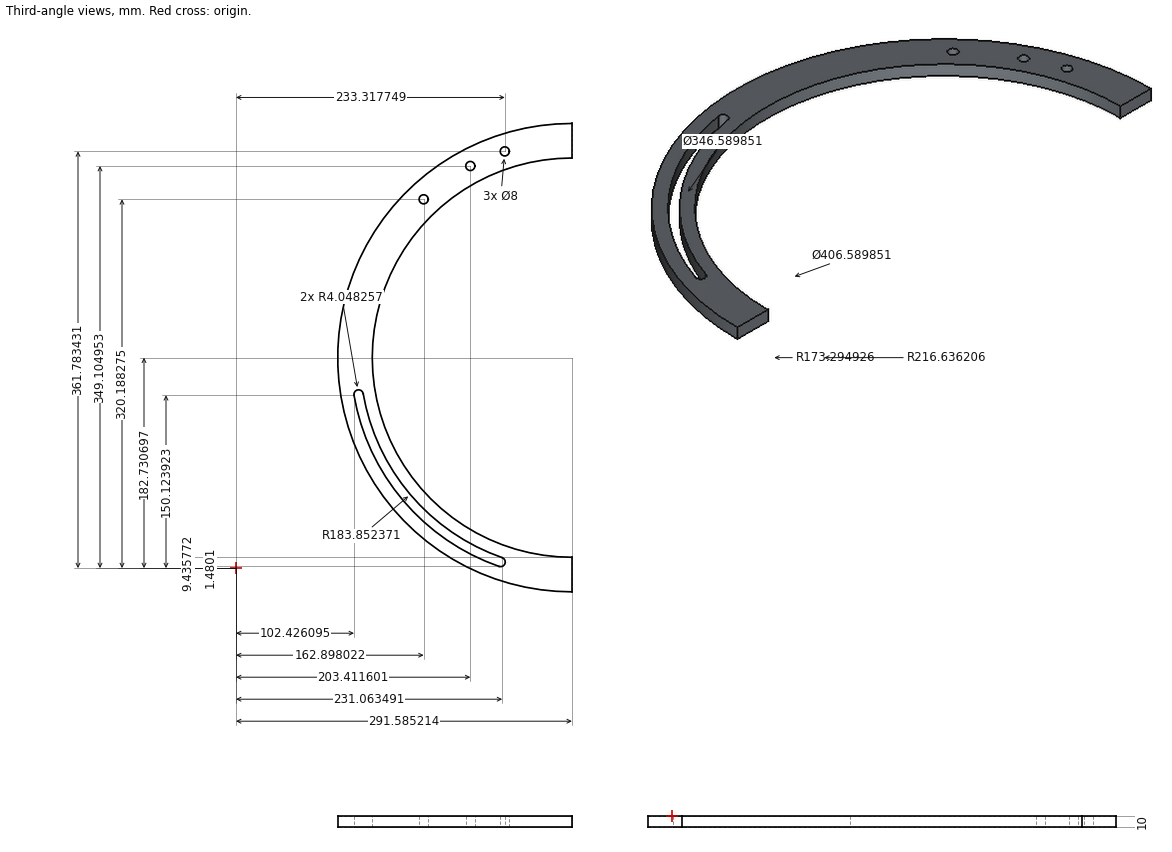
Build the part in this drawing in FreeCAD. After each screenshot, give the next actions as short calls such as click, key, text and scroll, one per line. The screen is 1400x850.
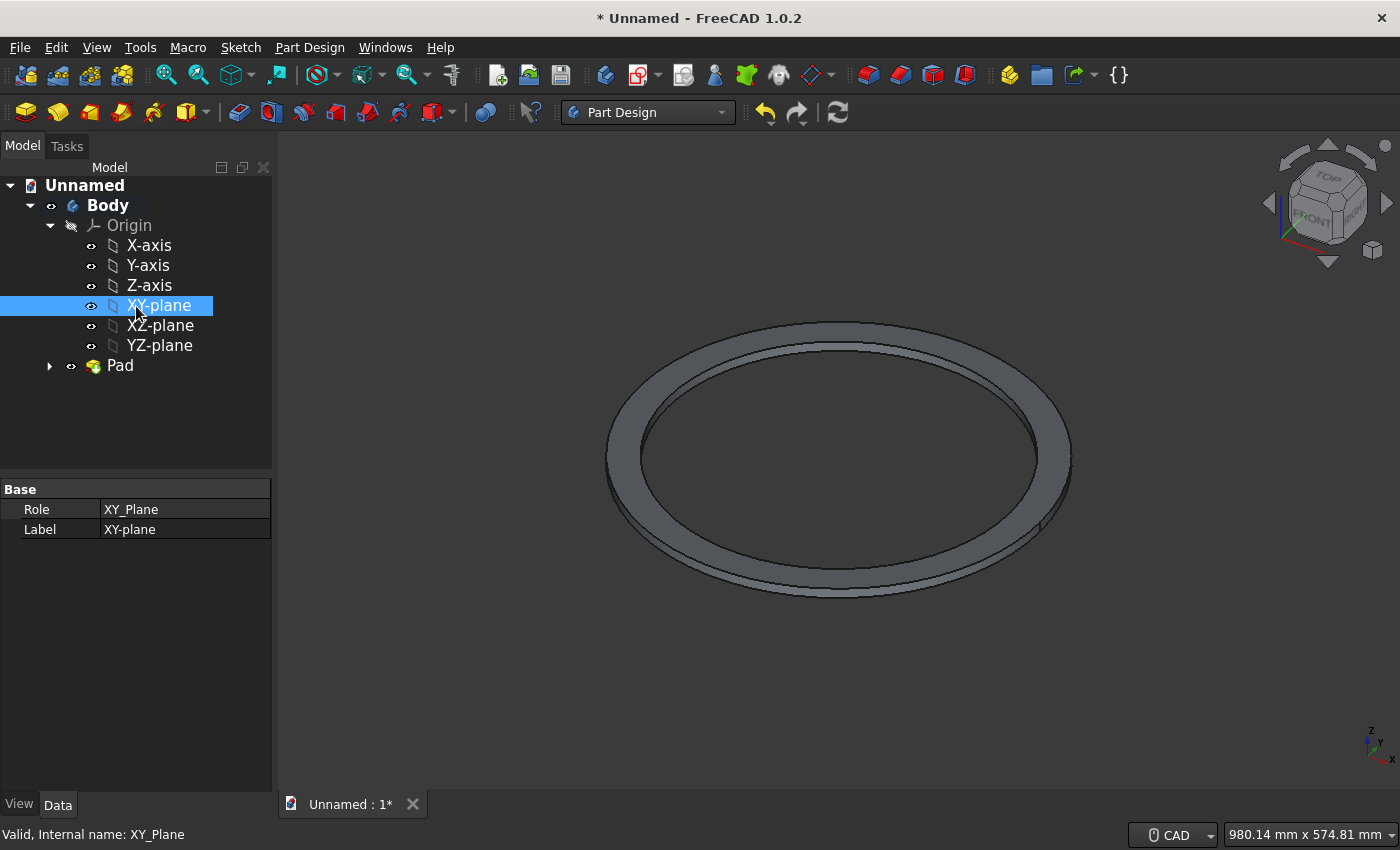
click(812, 76)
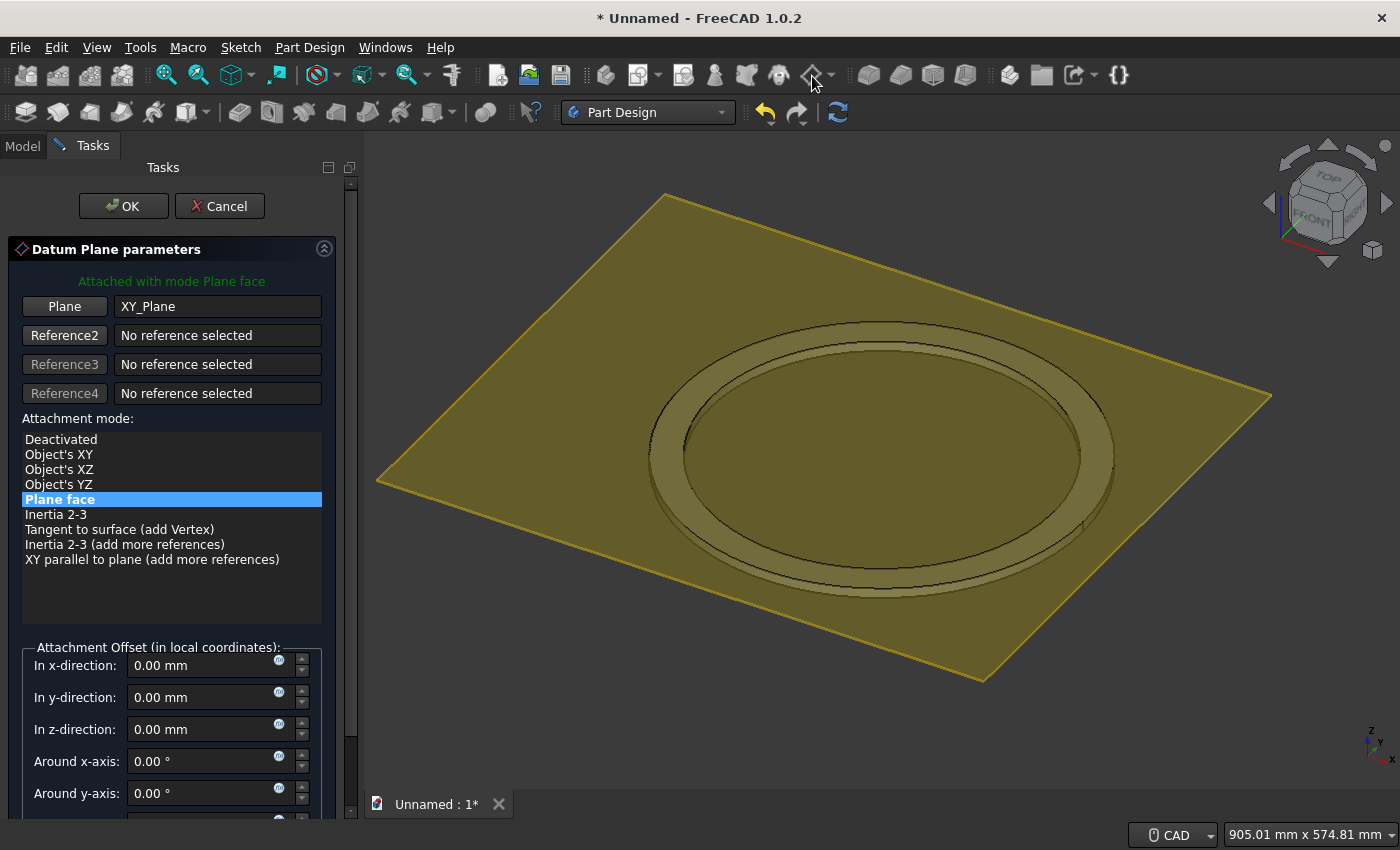
triple_click(210, 729)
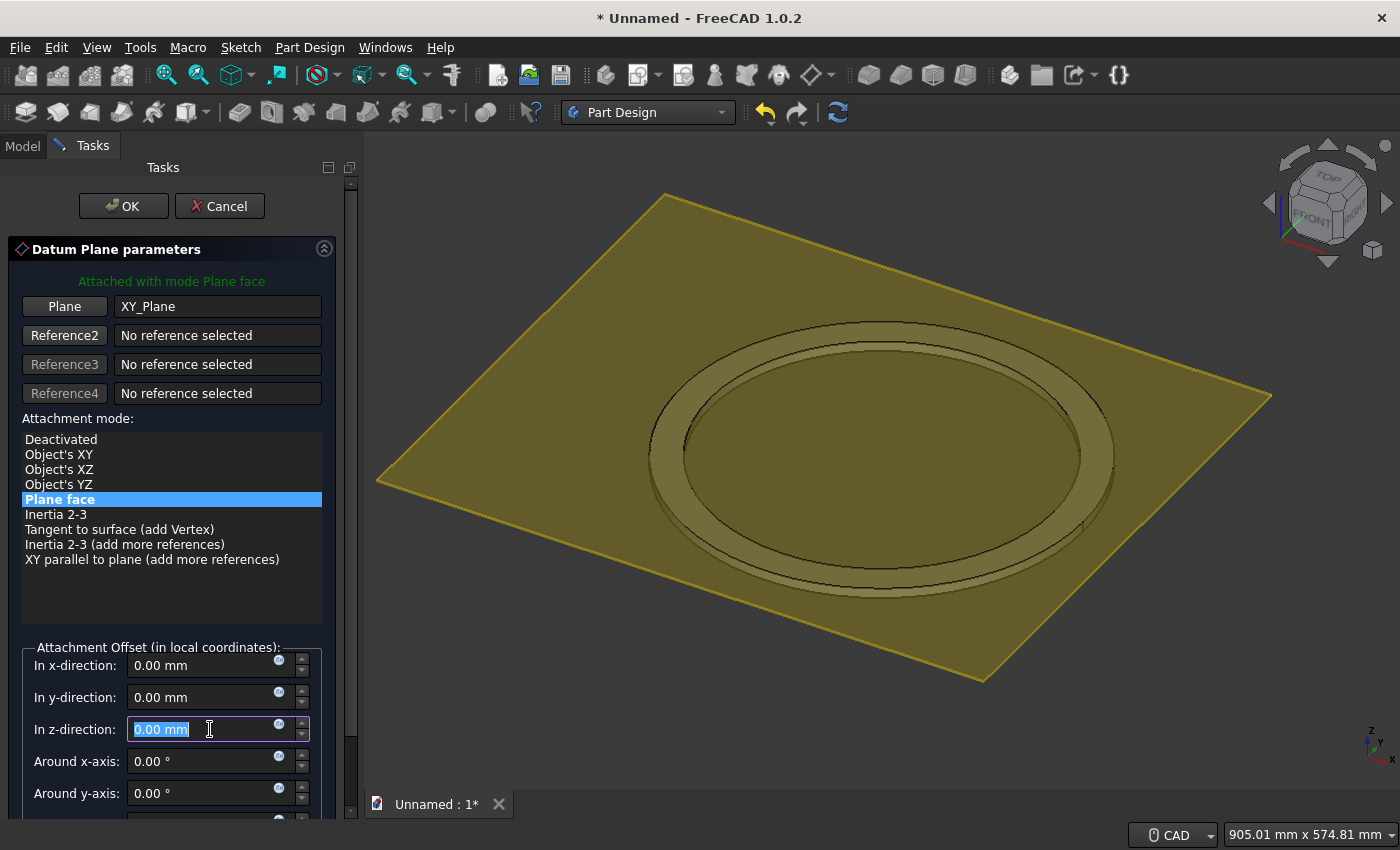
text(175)
key(Tab)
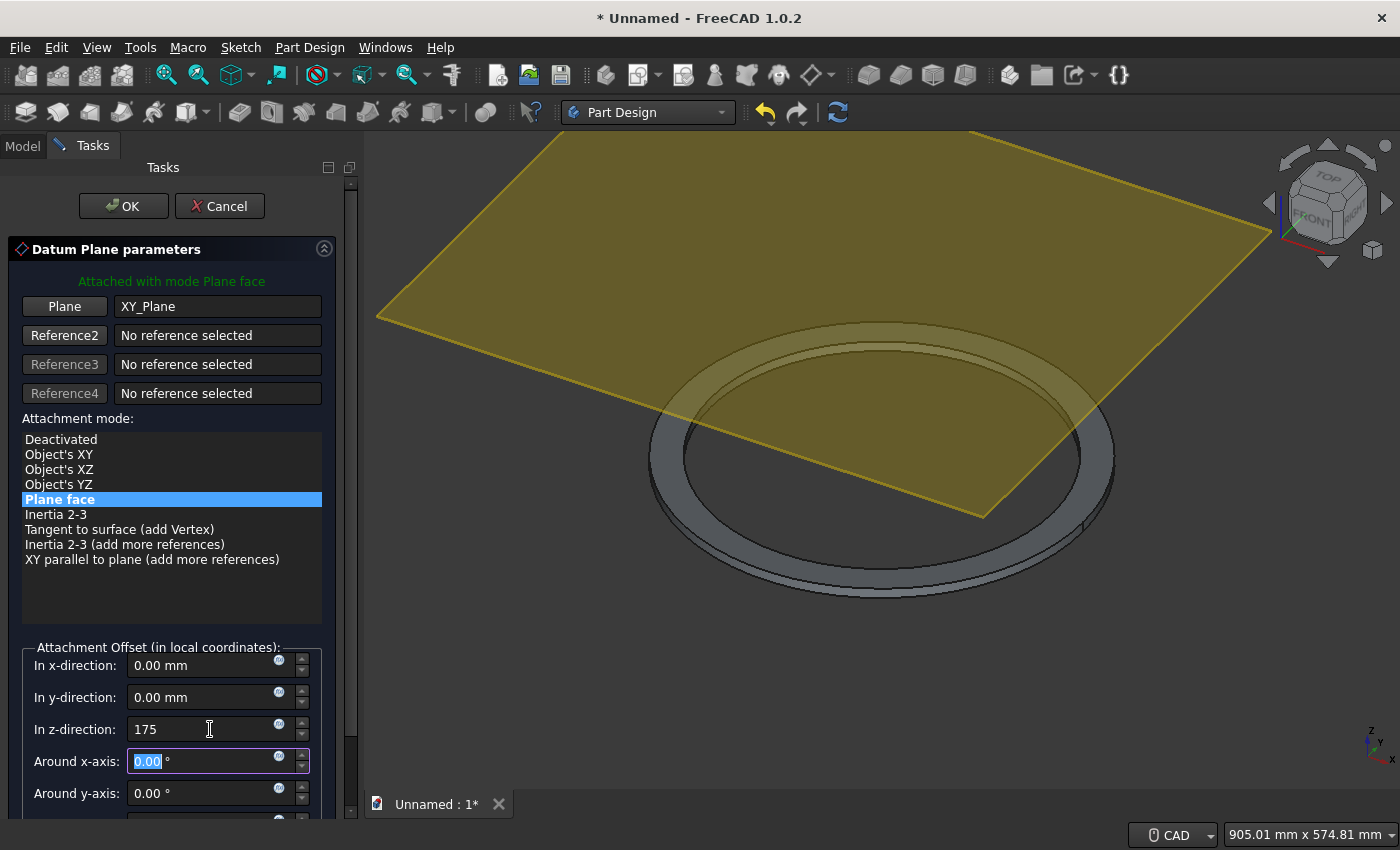
click(124, 206)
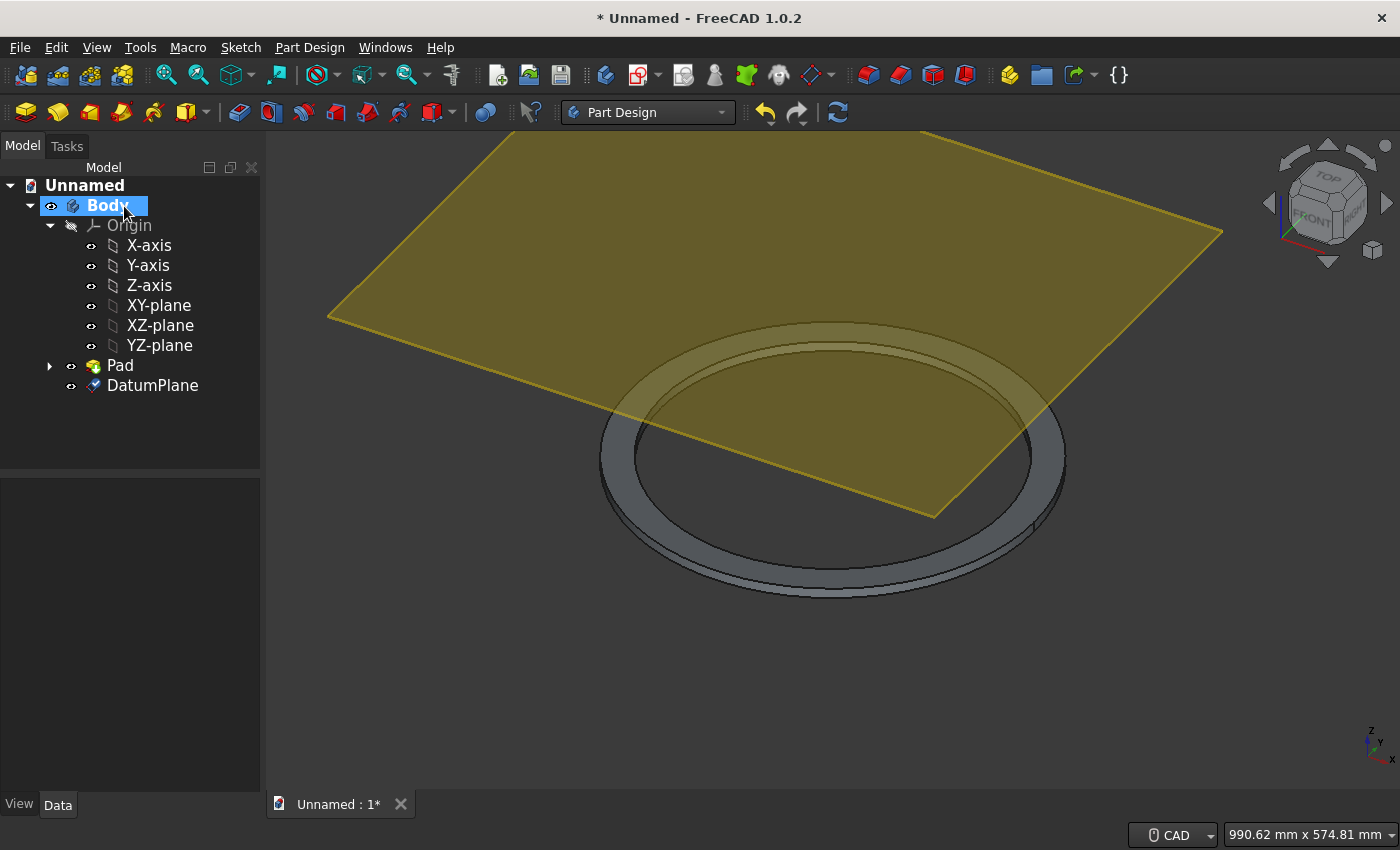
click(116, 386)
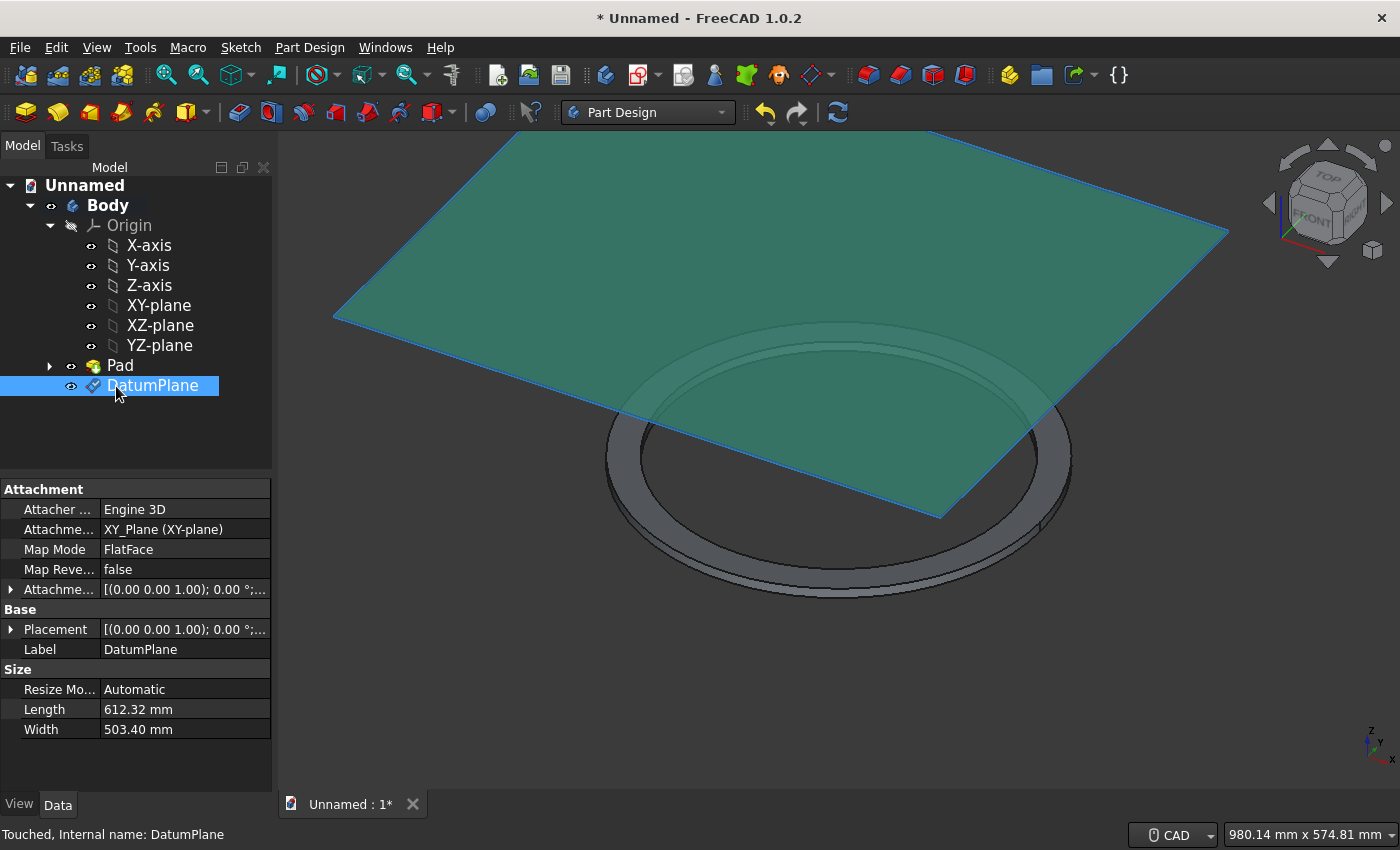
click(638, 76)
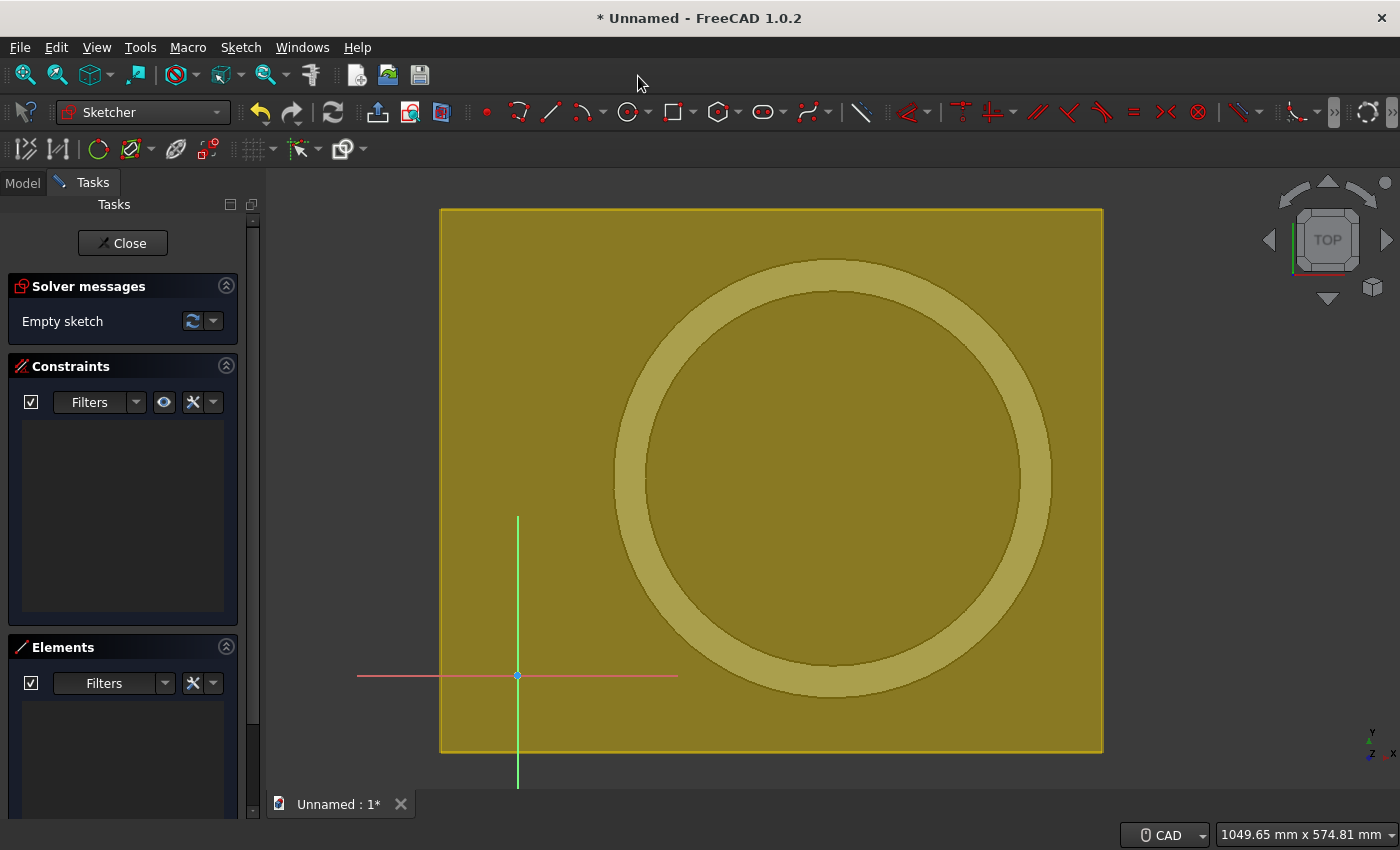
click(552, 112)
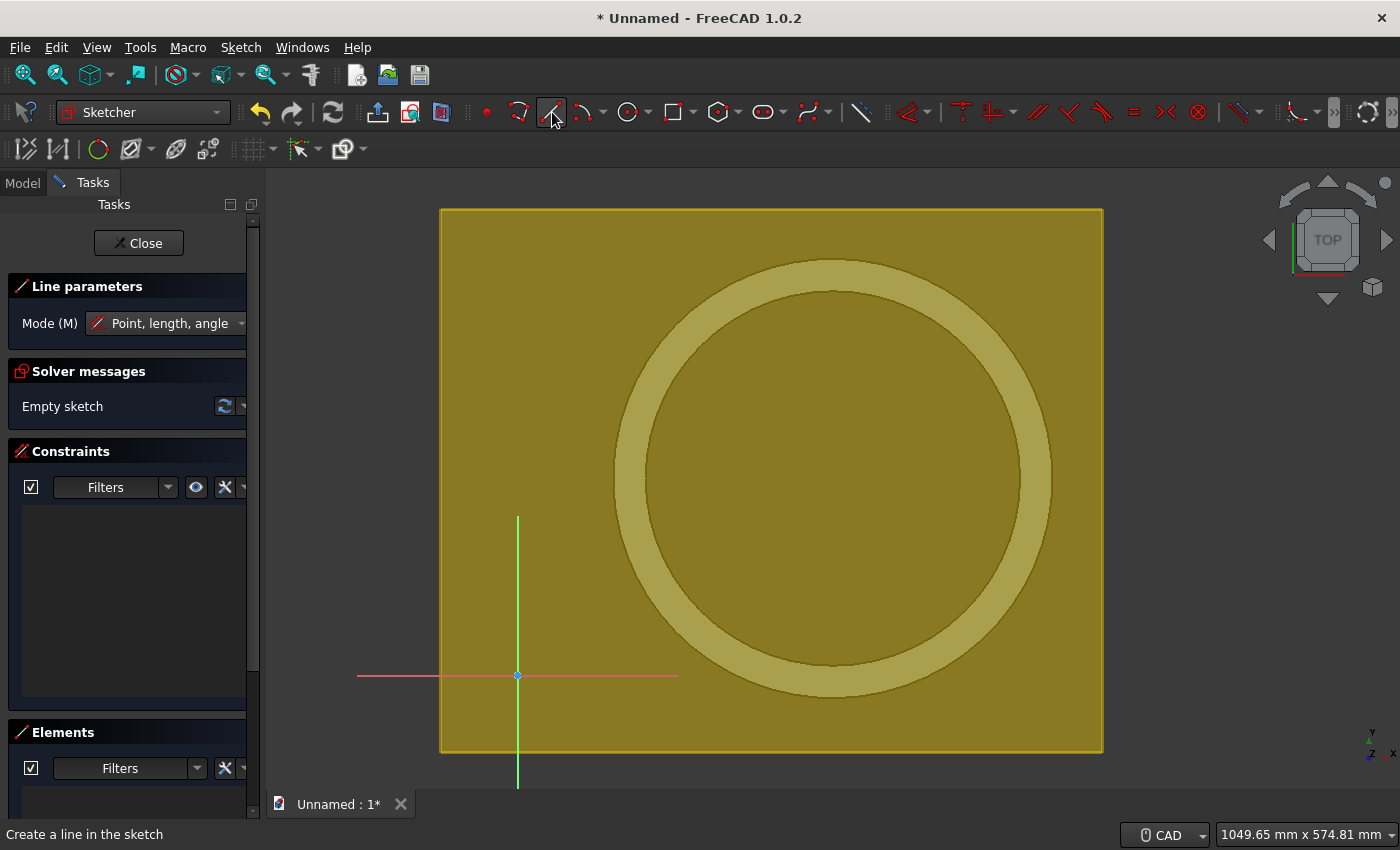
click(833, 713)